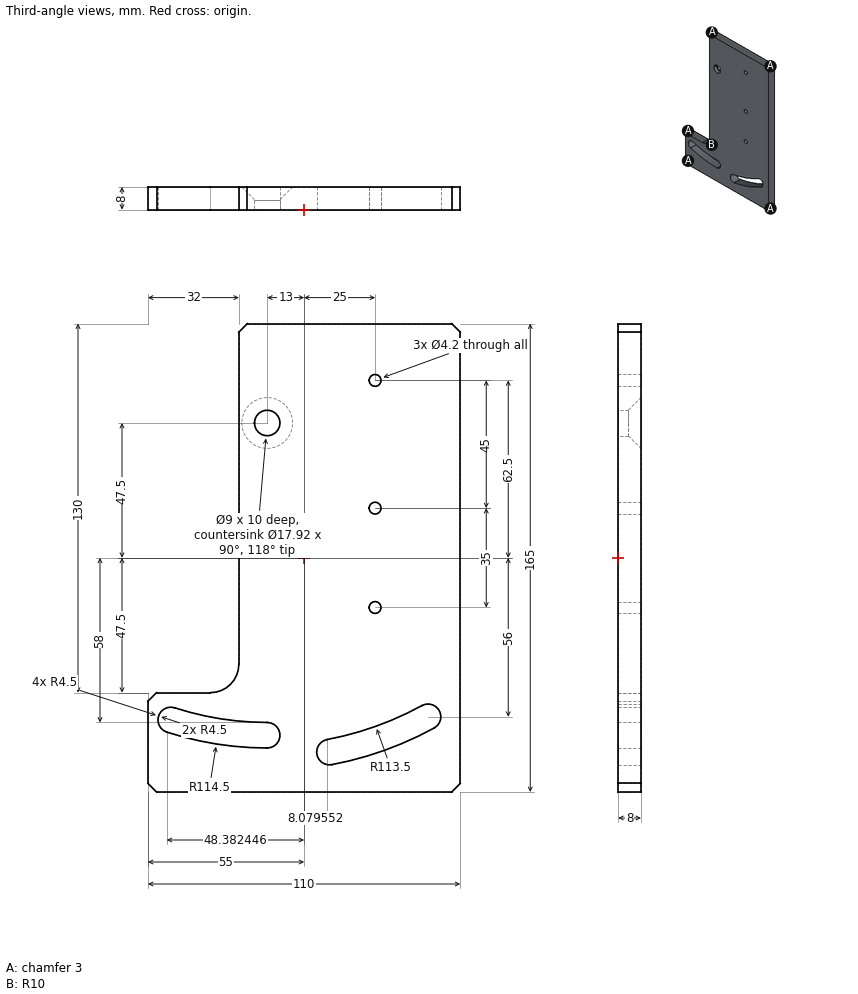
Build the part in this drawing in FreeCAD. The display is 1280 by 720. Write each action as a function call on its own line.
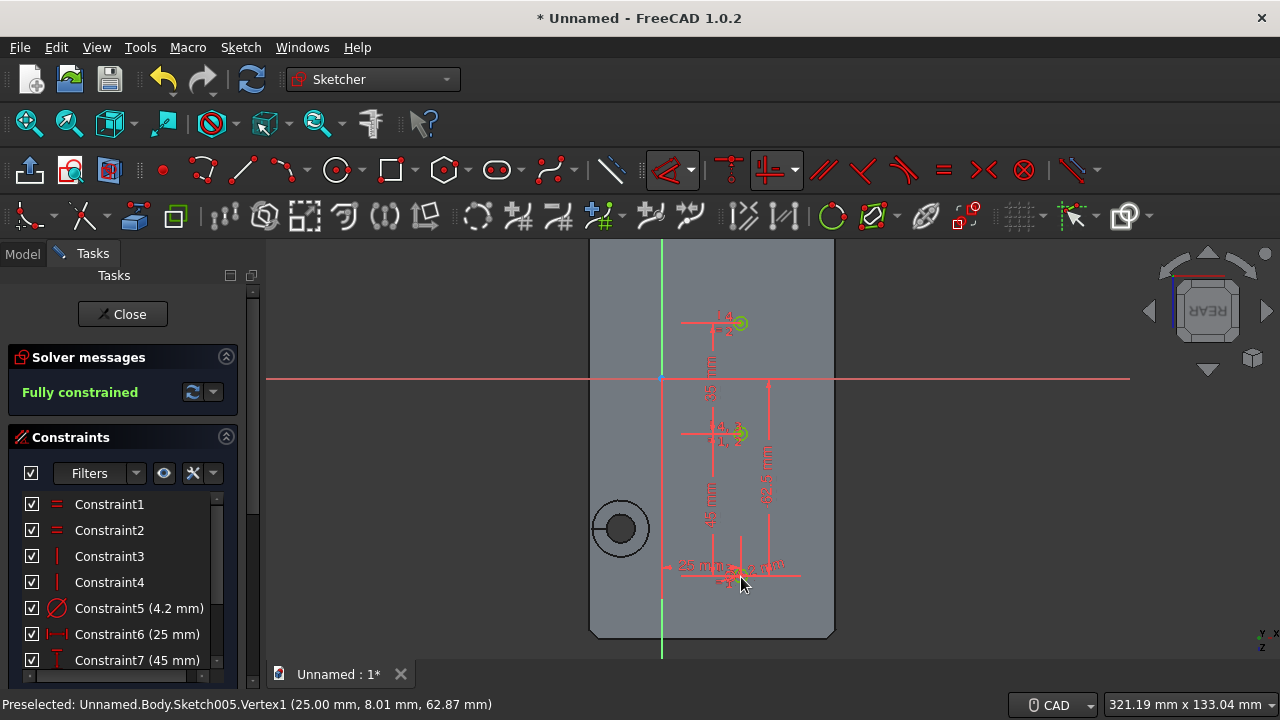
click(123, 314)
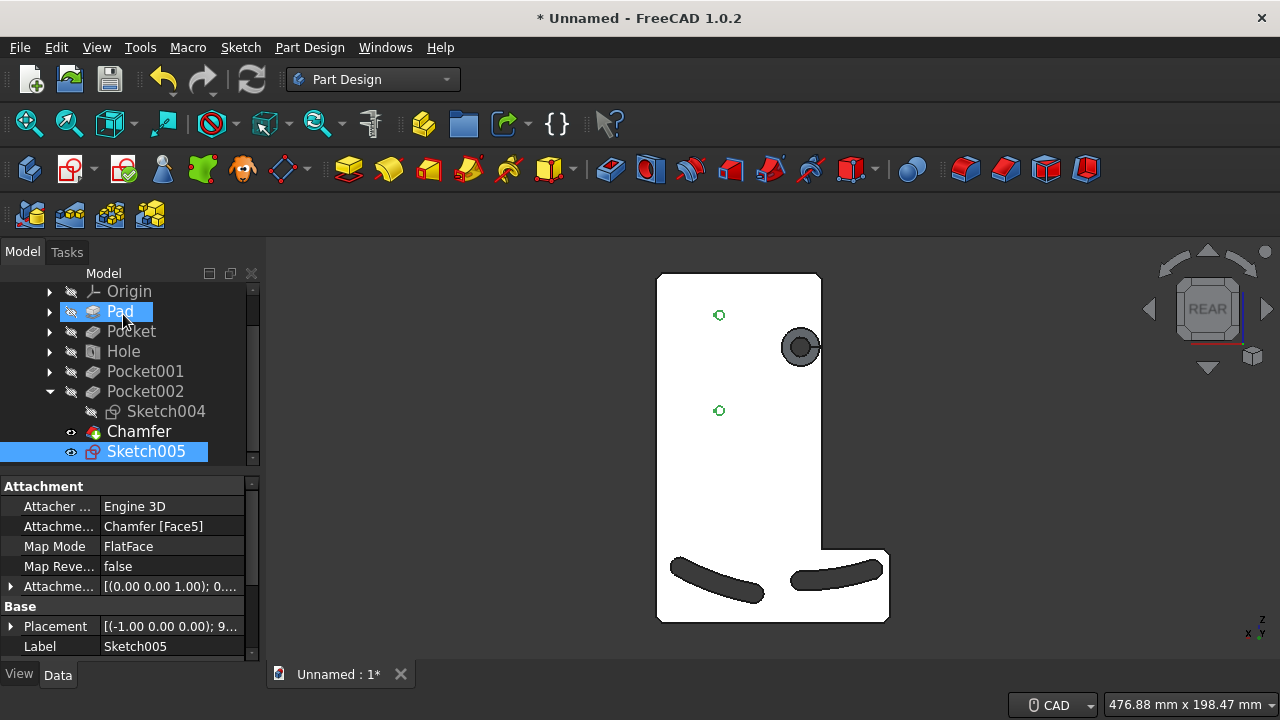
click(652, 170)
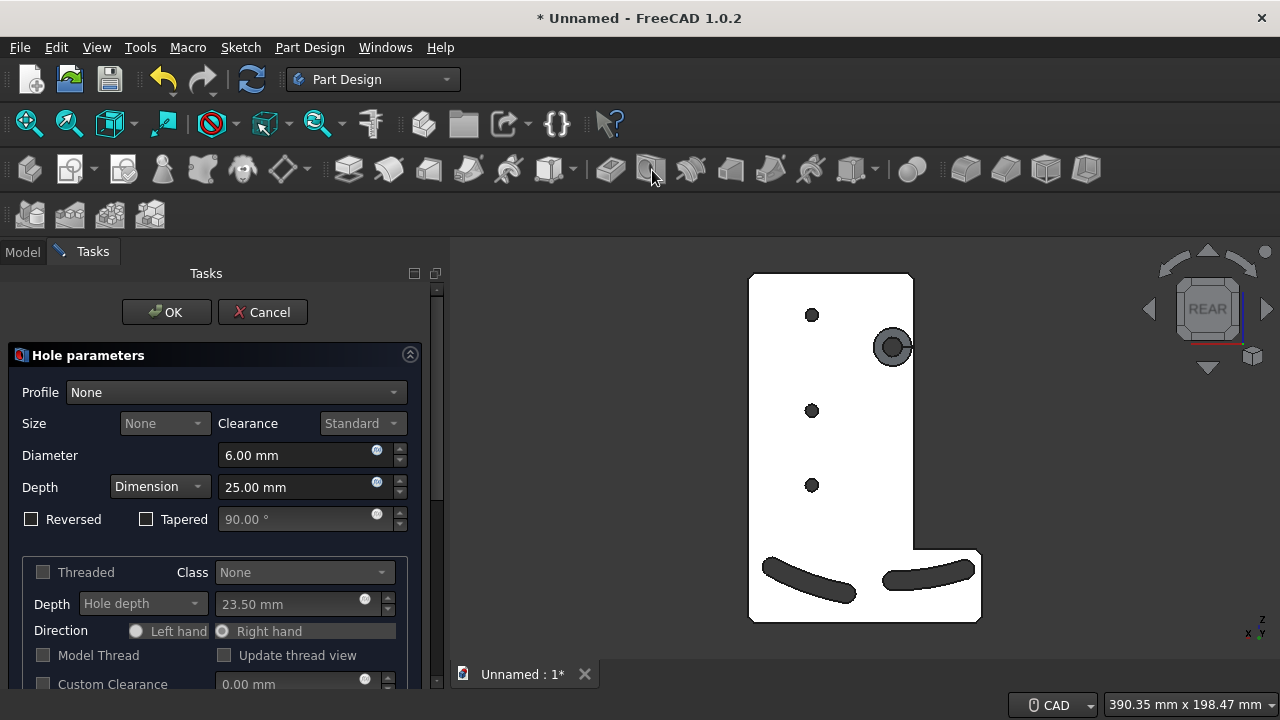
triple_click(305, 455)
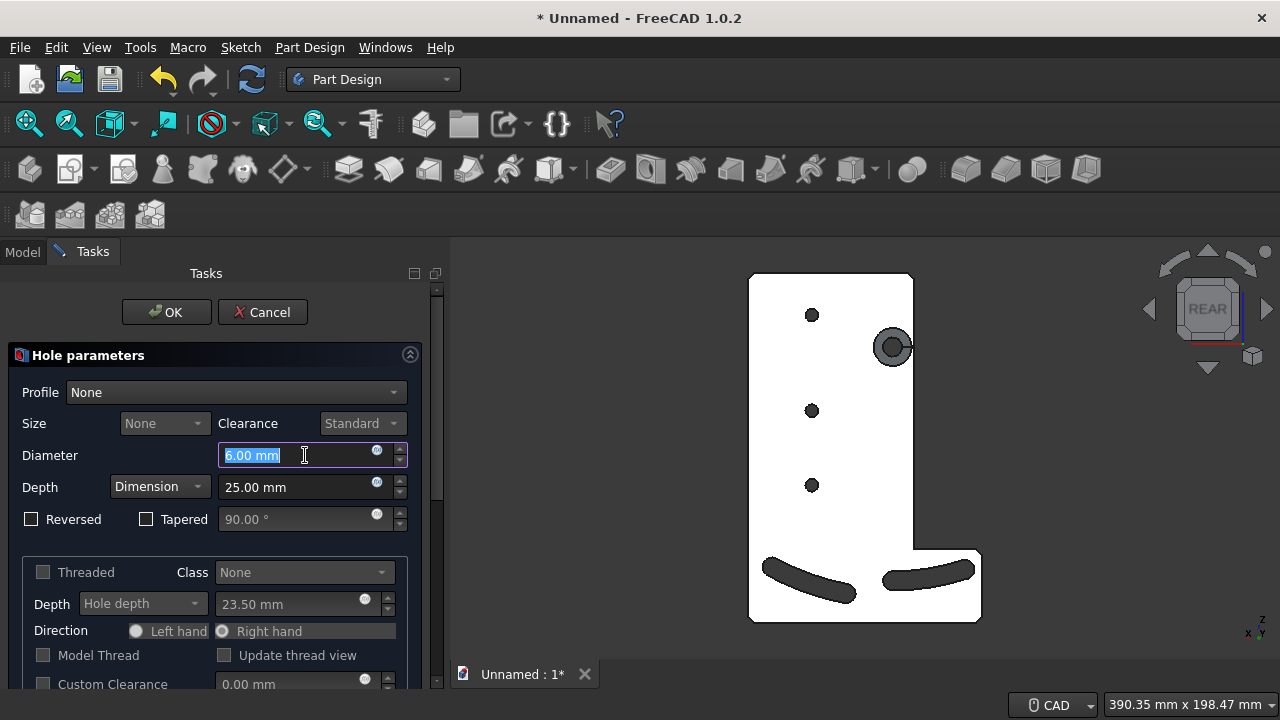
text(4.2)
key(Tab)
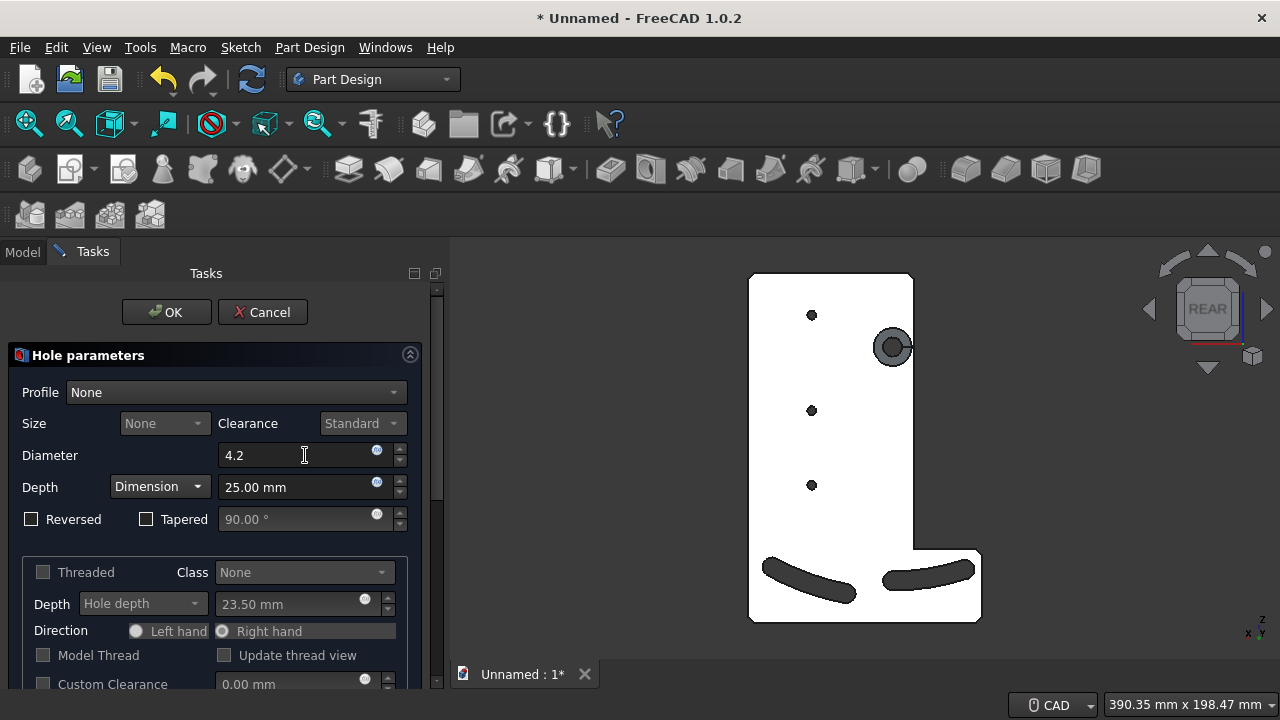
click(161, 486)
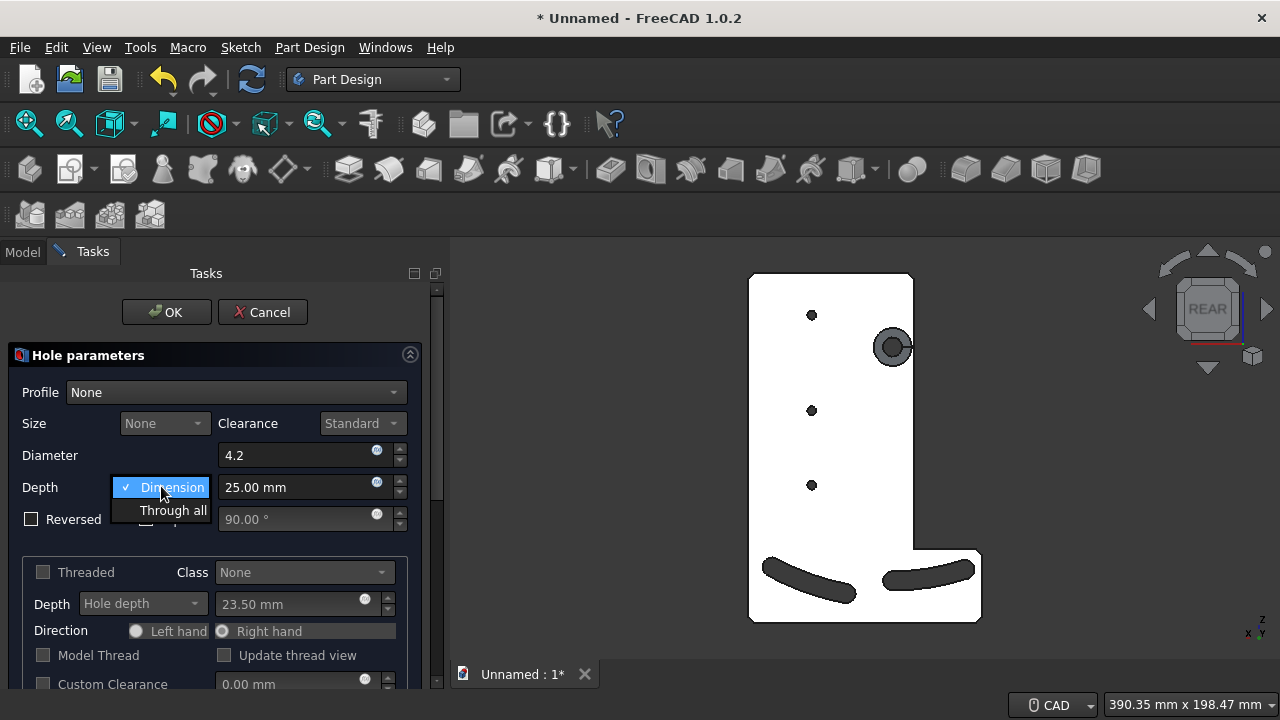
click(160, 510)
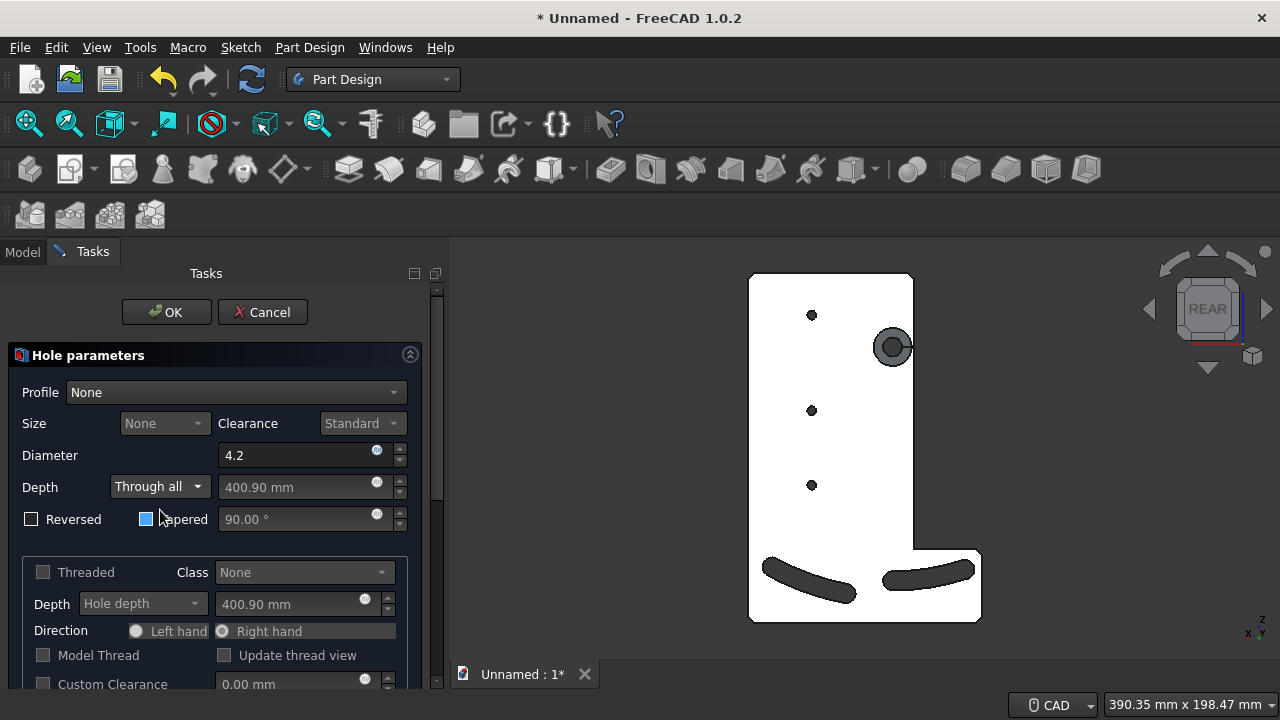
click(167, 312)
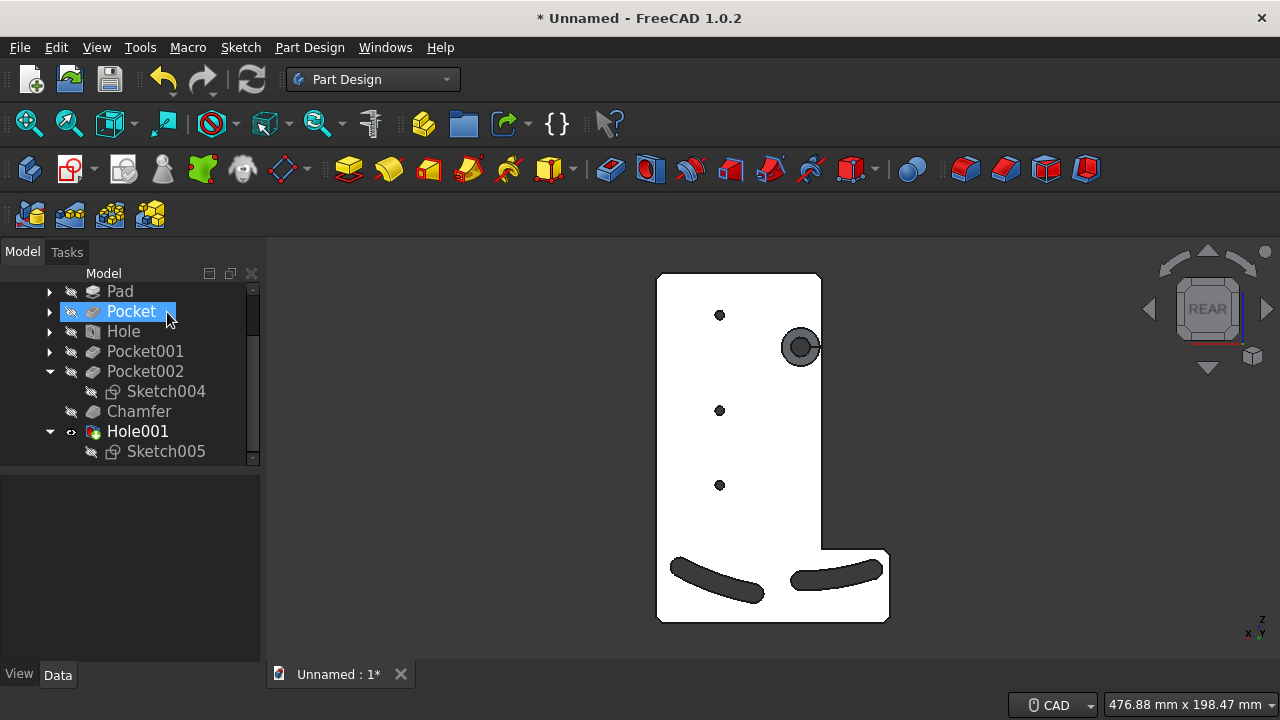
scroll(822, 548, up, 5)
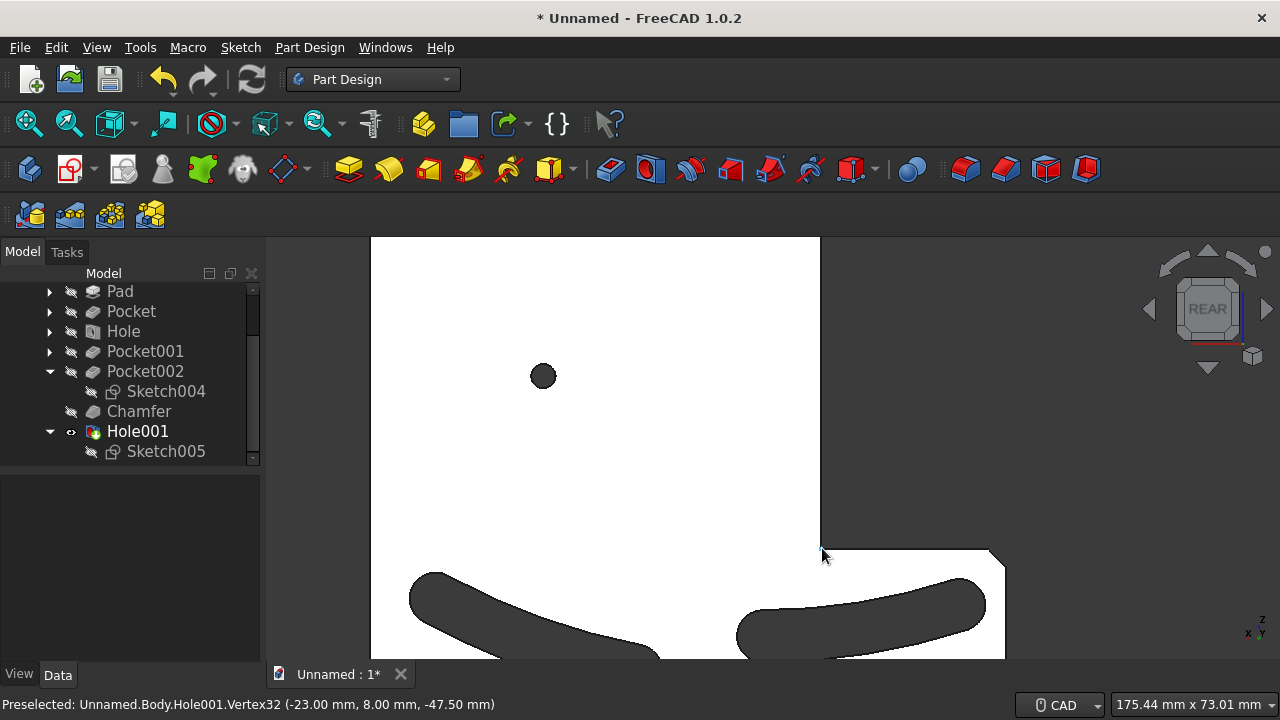
click(30, 124)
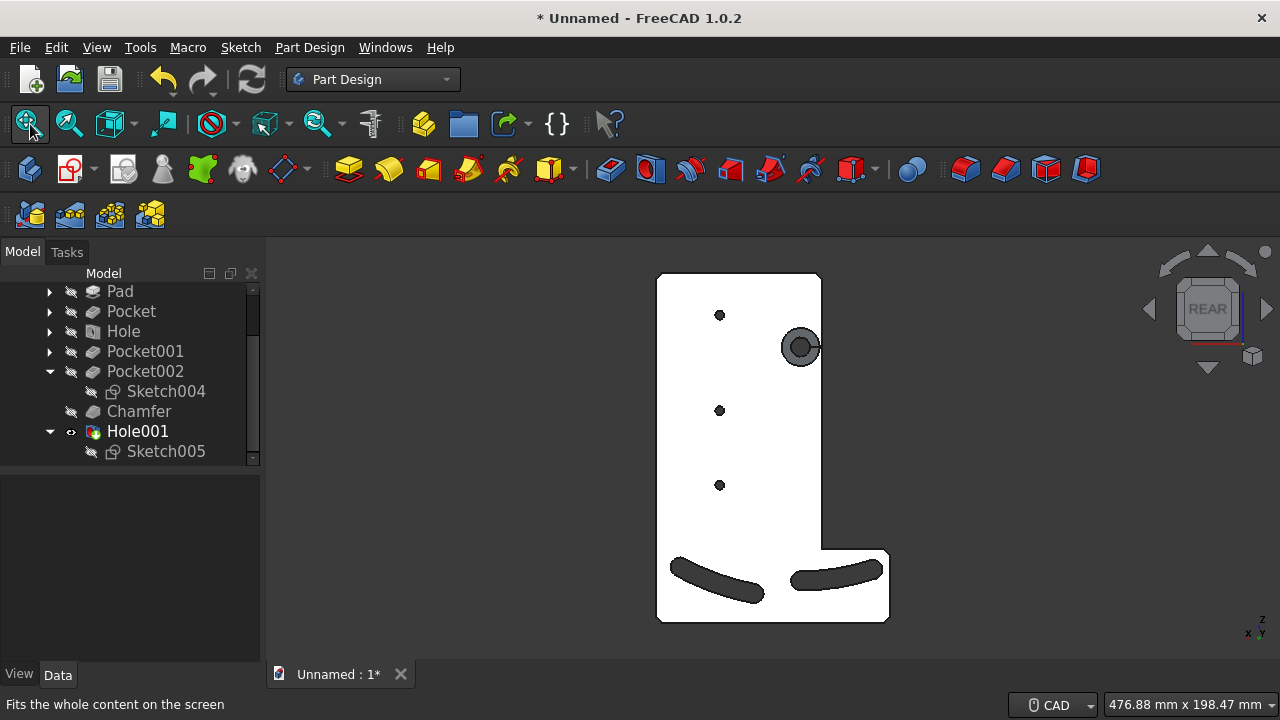
key(0)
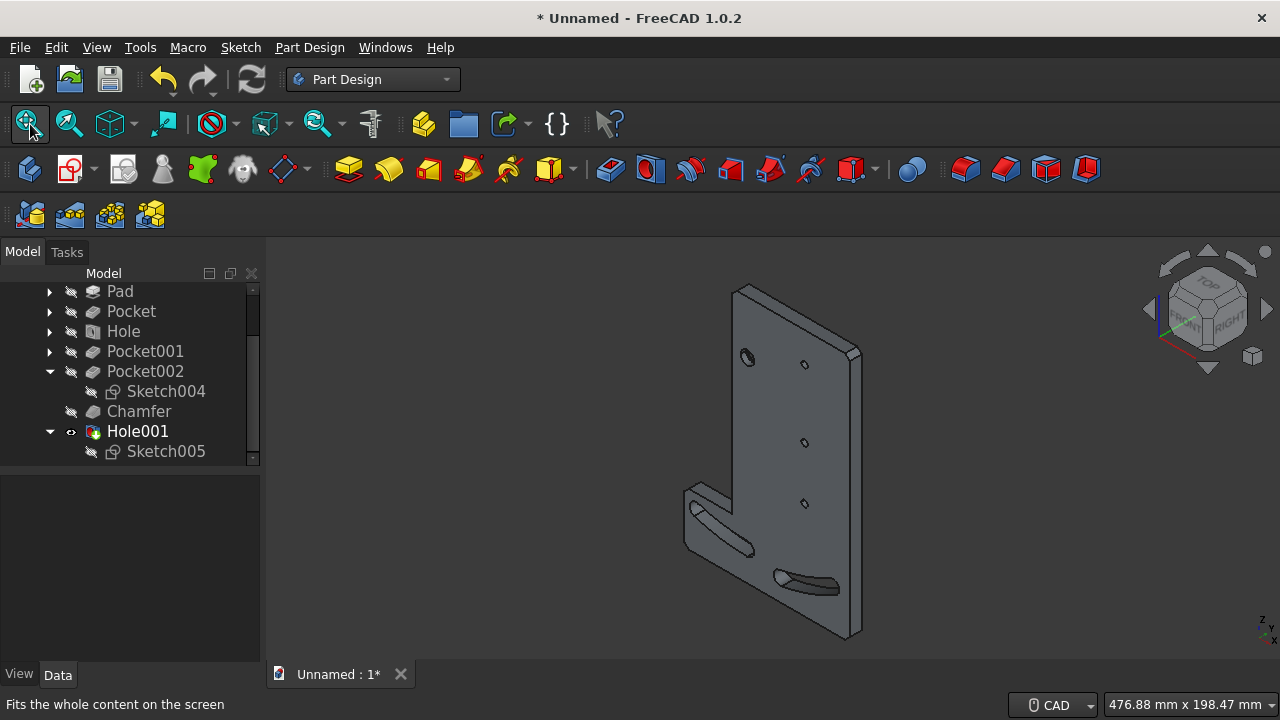
scroll(738, 510, up, 5)